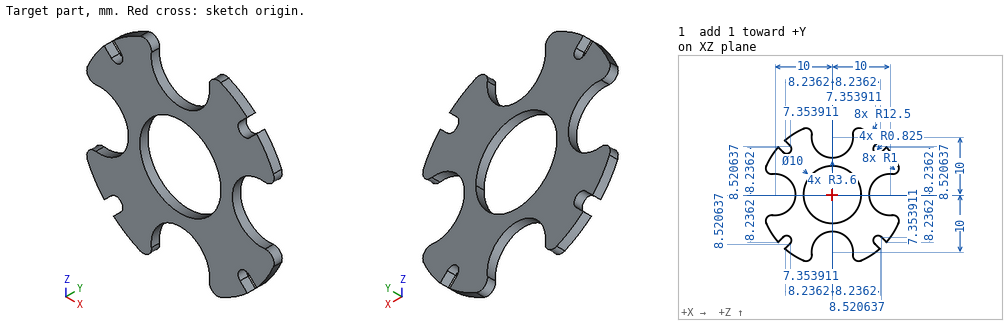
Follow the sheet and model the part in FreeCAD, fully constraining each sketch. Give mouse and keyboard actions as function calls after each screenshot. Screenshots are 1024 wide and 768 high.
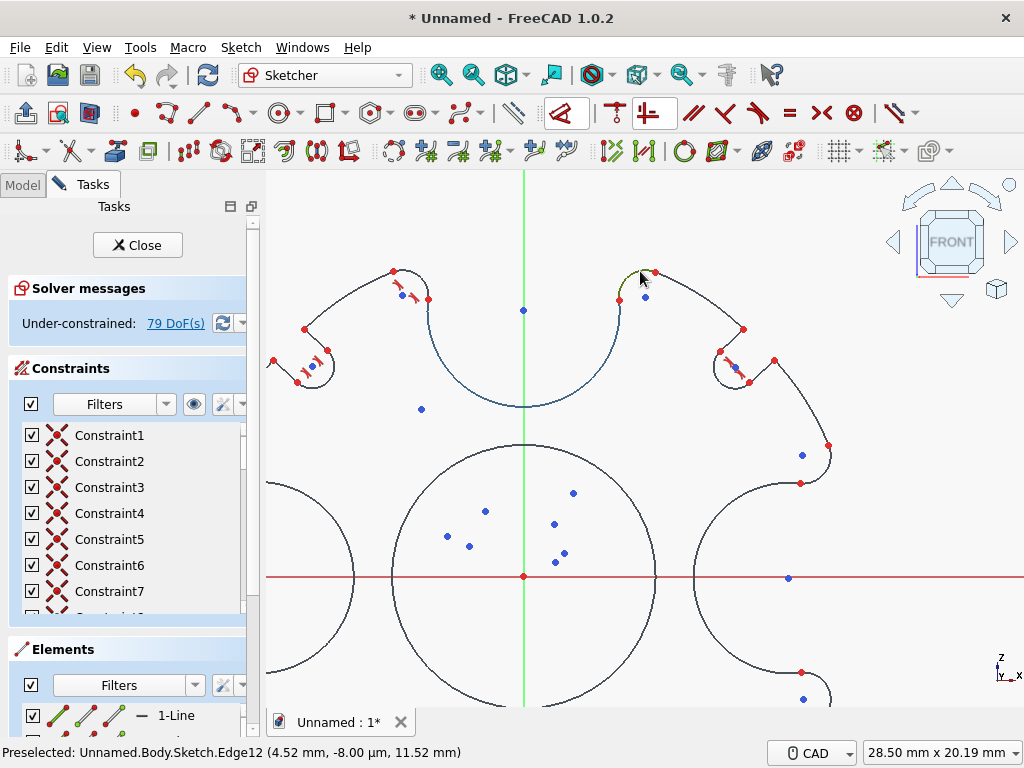
click(758, 114)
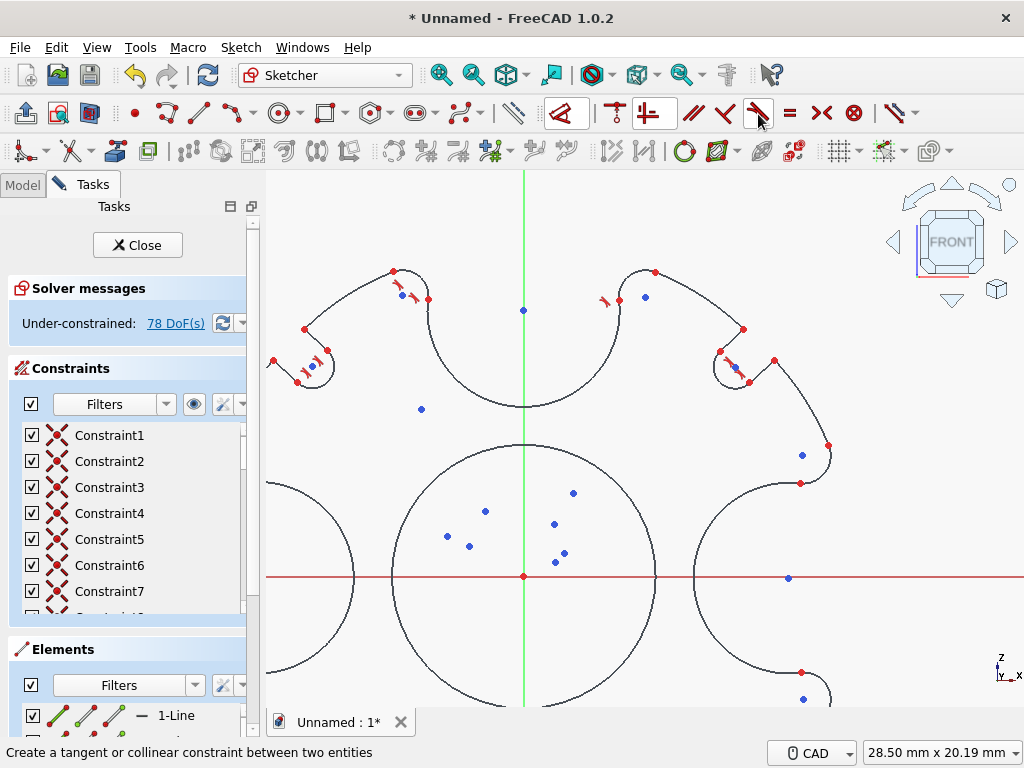
click(640, 271)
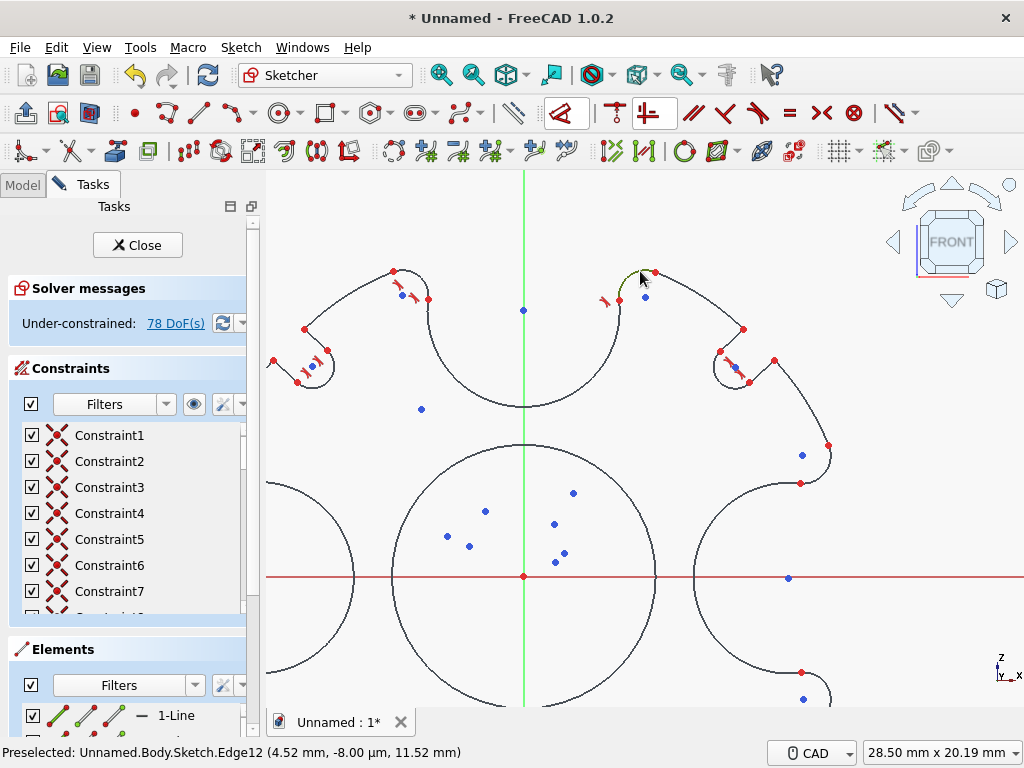
click(720, 309)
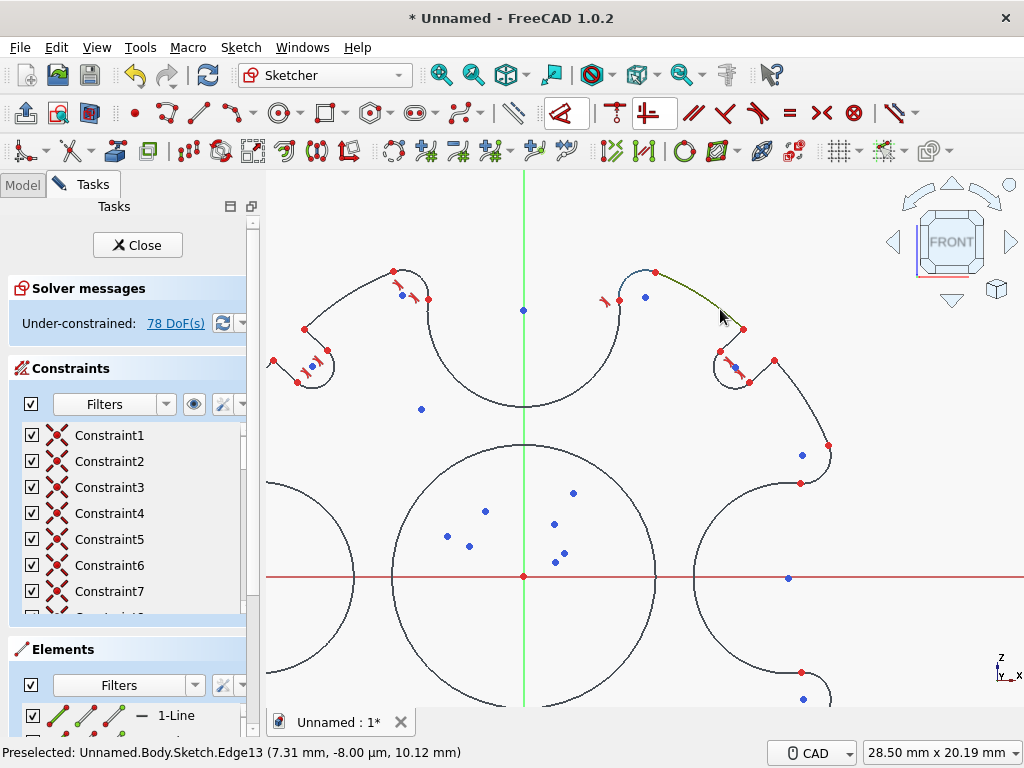
key(t)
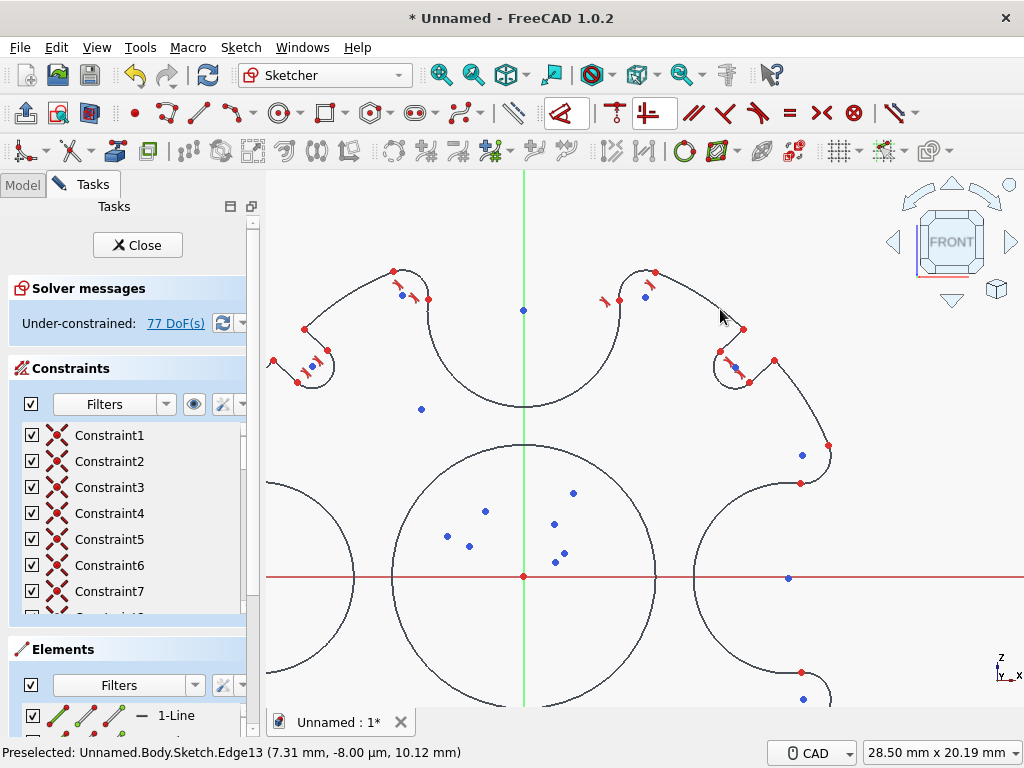
click(816, 418)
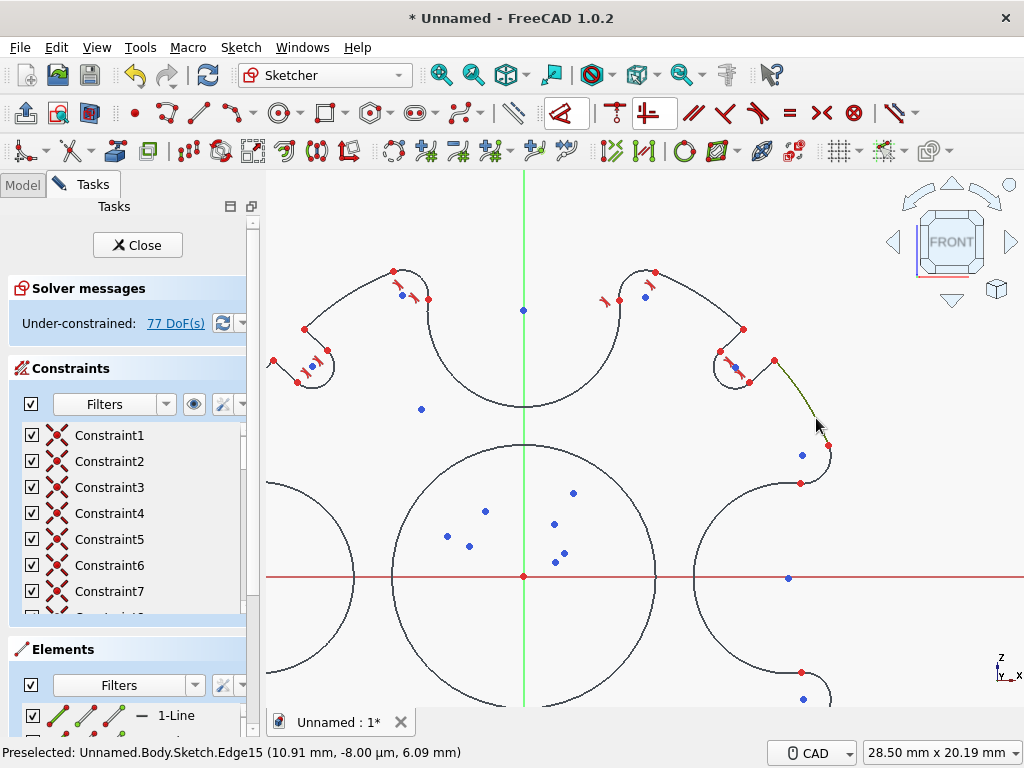
click(817, 480)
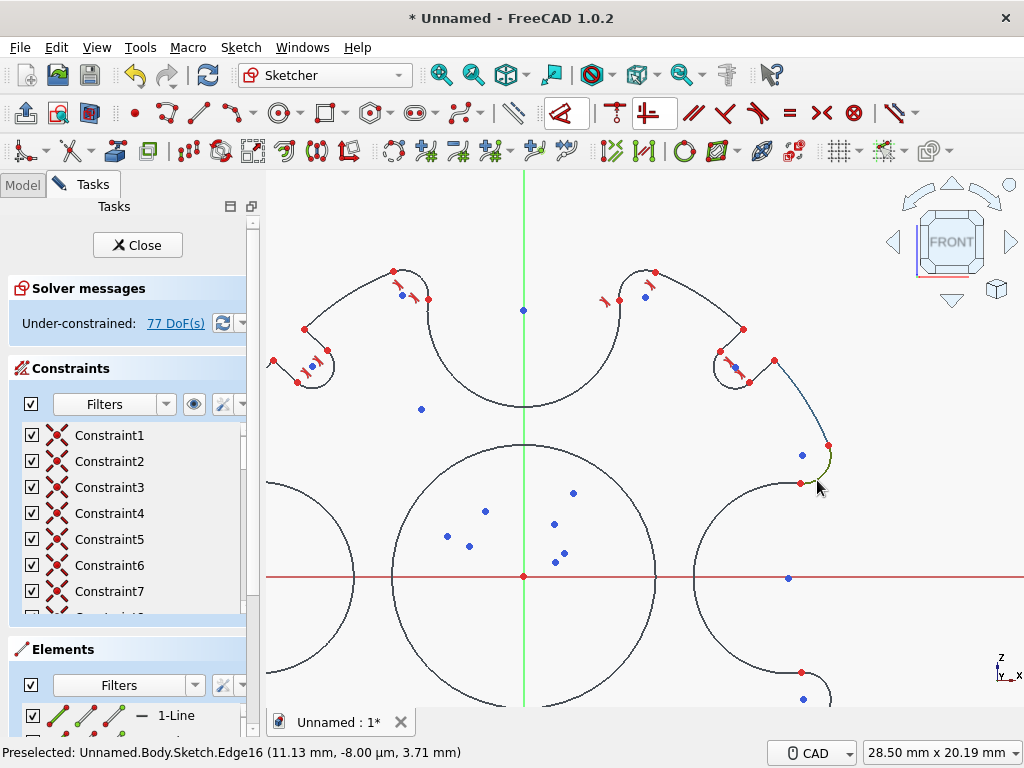
click(758, 114)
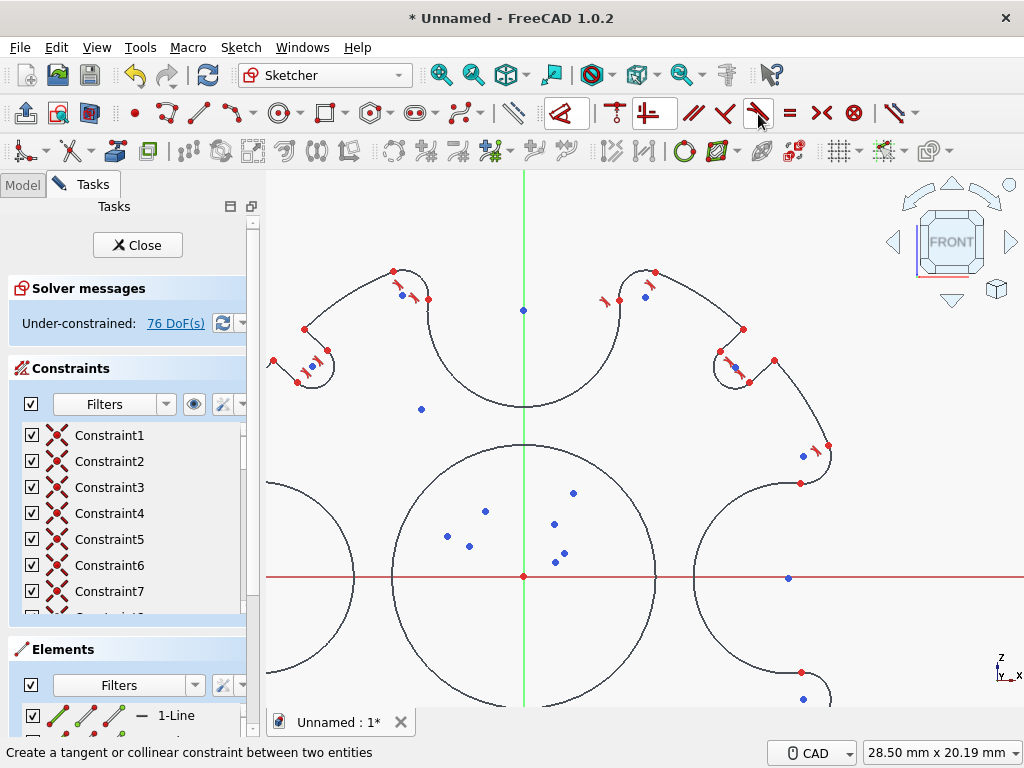
click(817, 480)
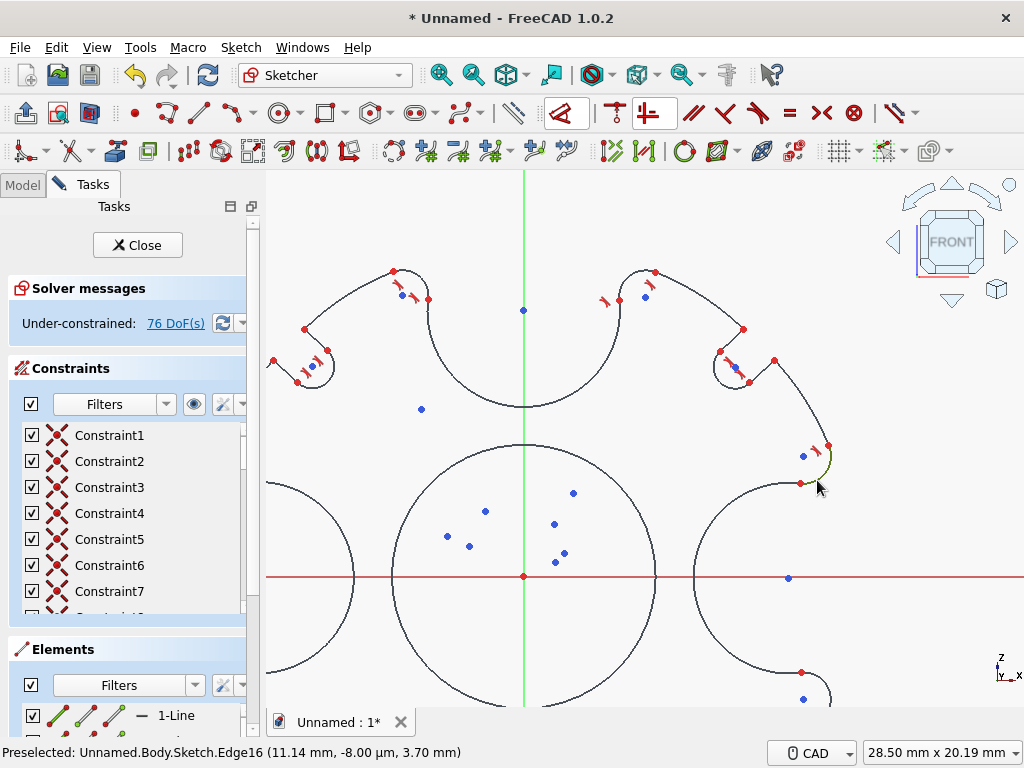
click(715, 518)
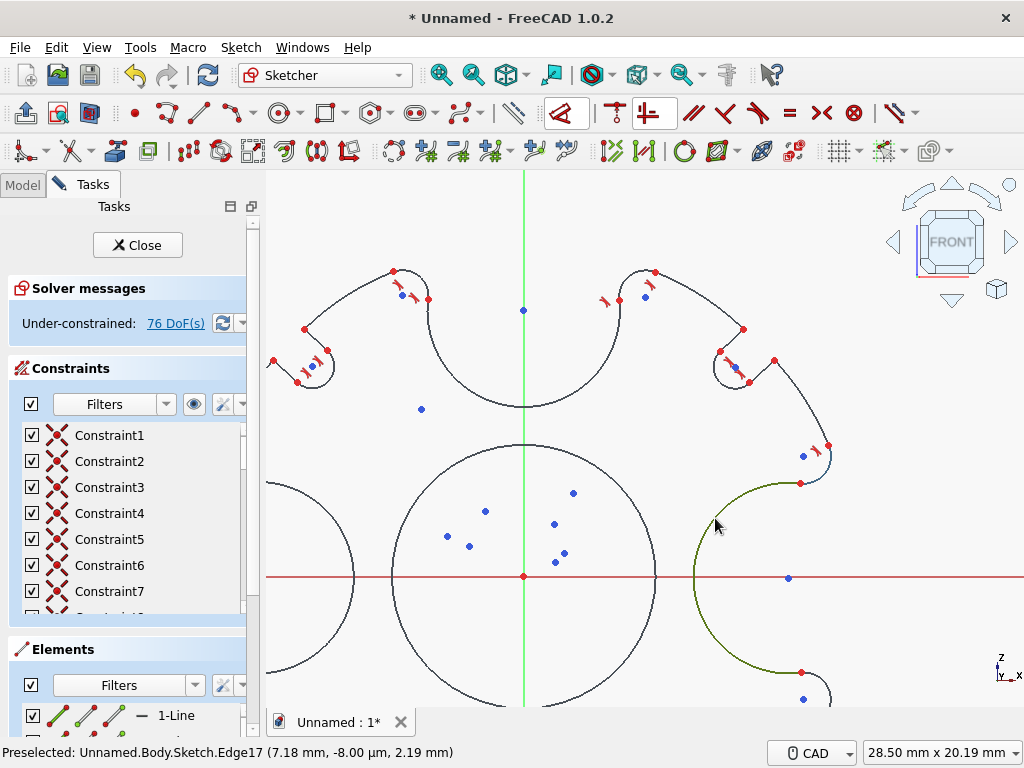
key(t)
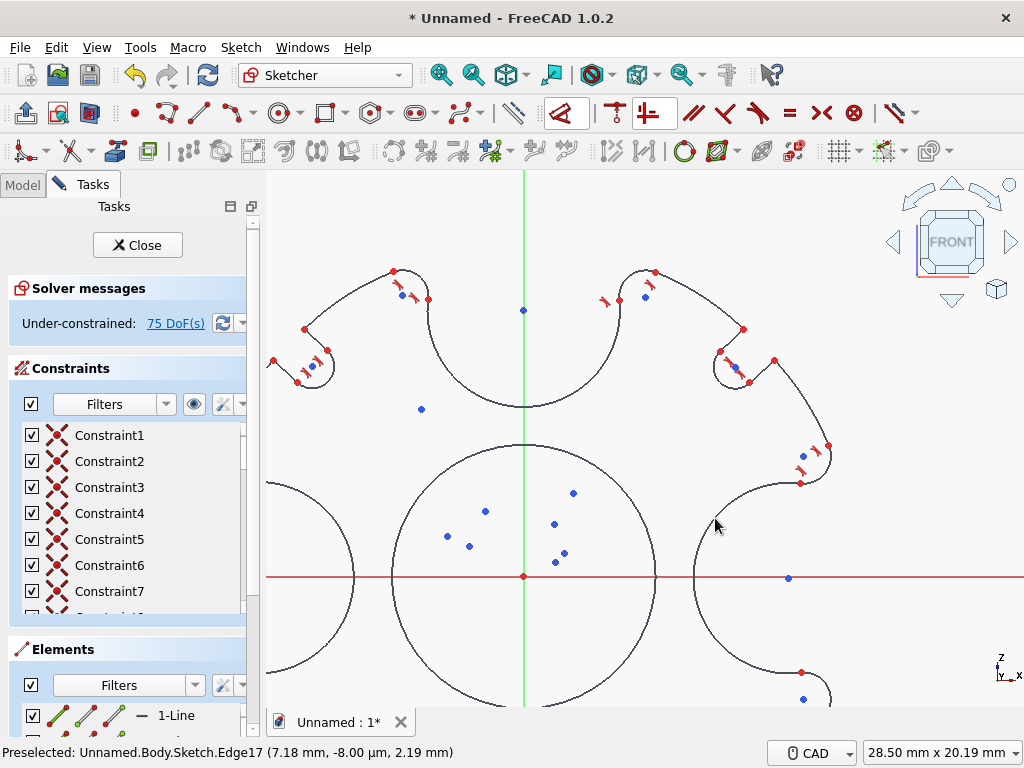
click(714, 519)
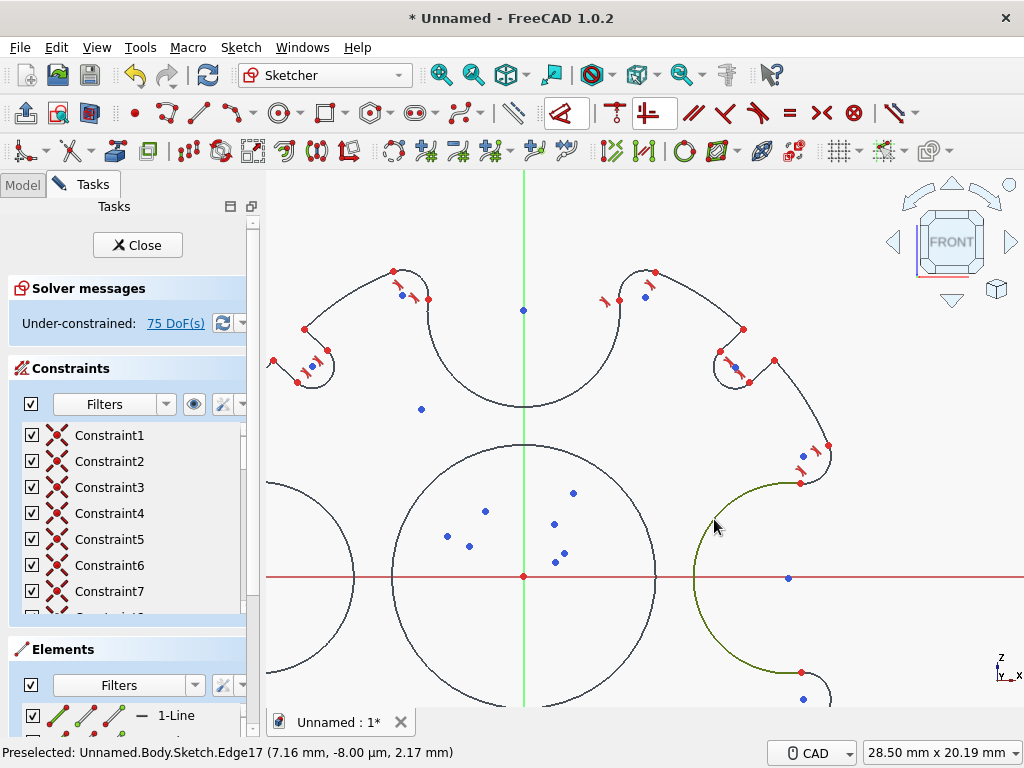
click(817, 676)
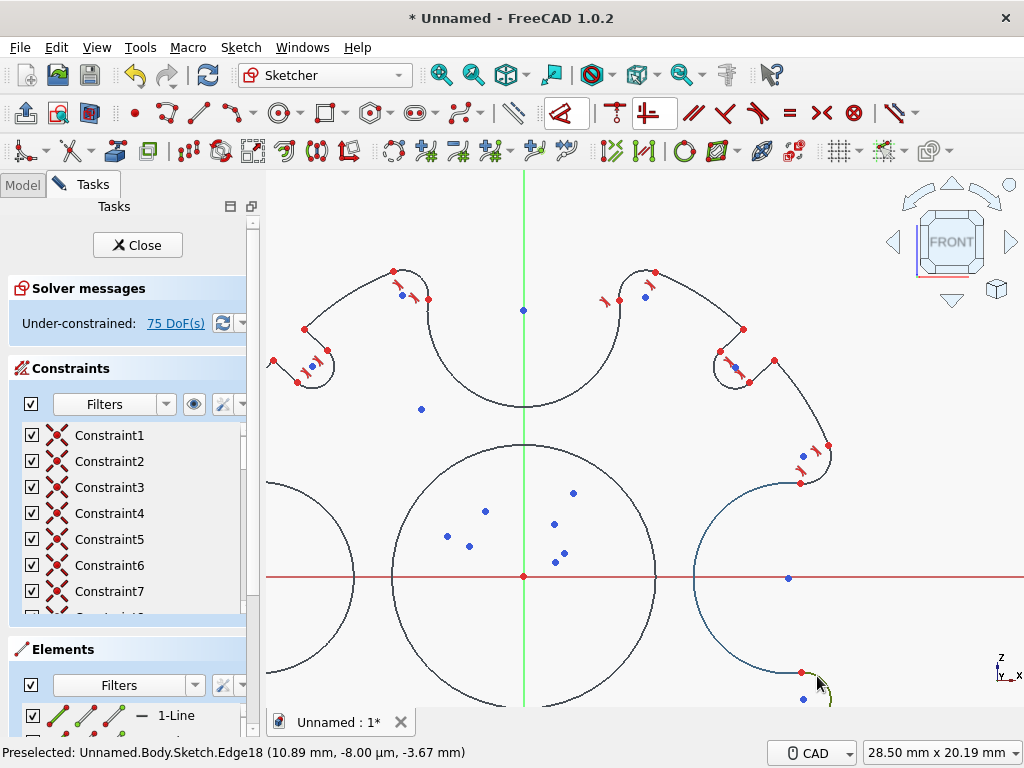
key(t)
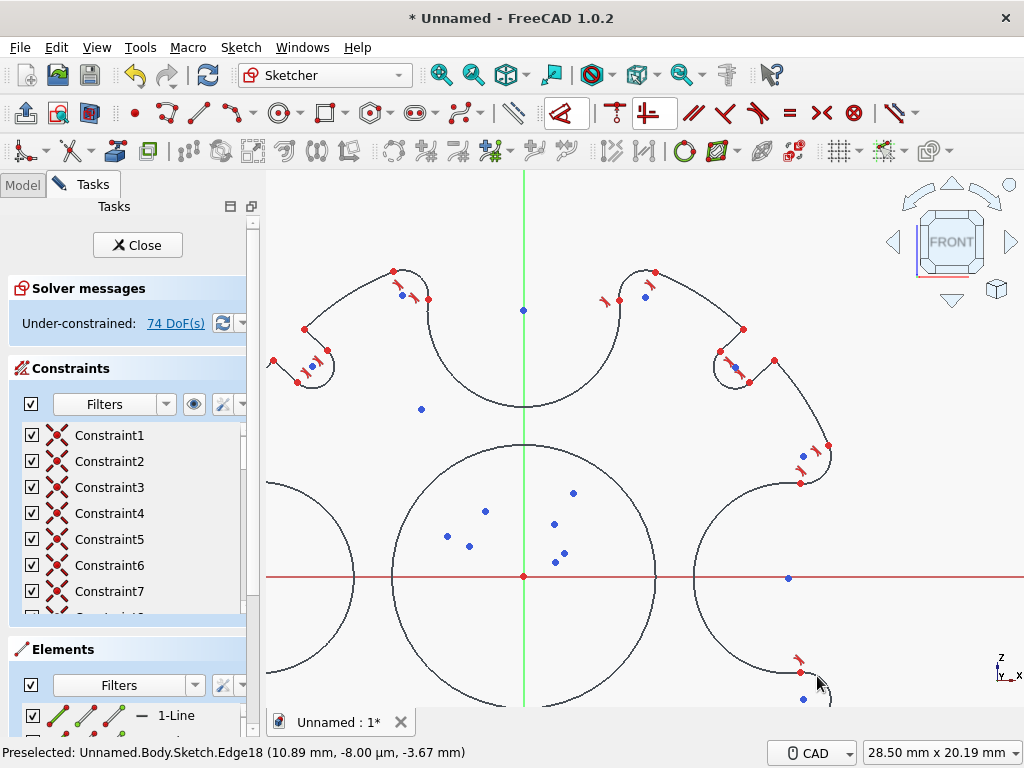
click(817, 676)